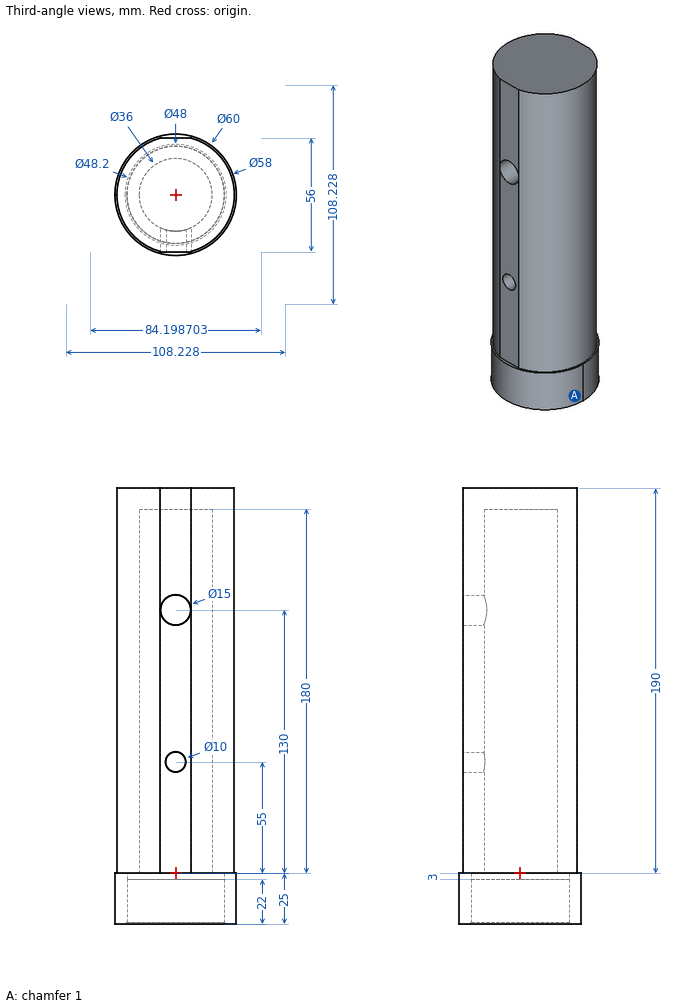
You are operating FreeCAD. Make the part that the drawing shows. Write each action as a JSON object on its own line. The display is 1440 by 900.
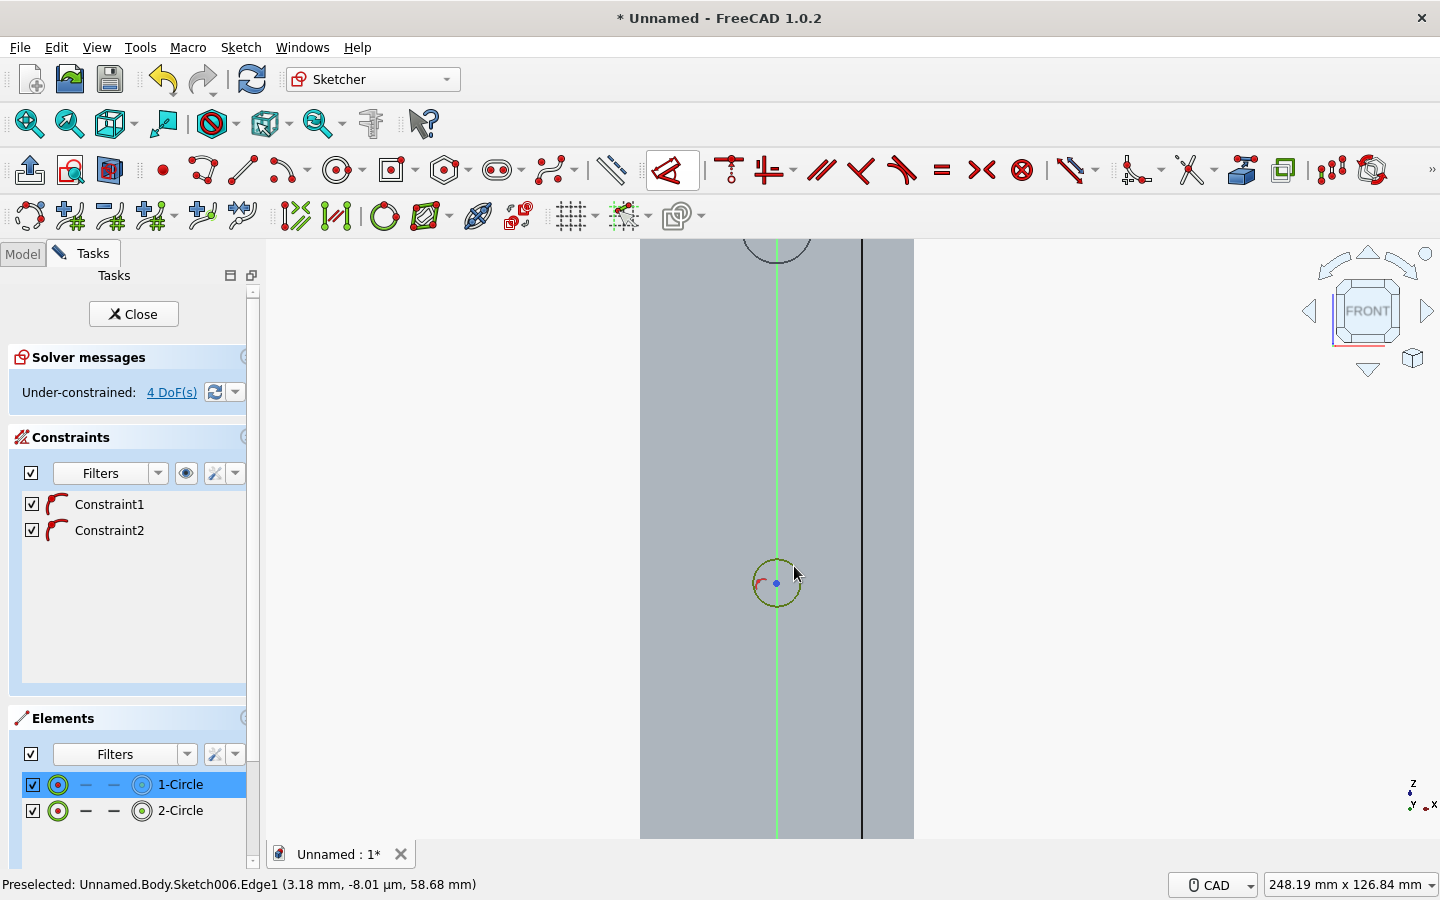
{"action": "key", "text": "k o"}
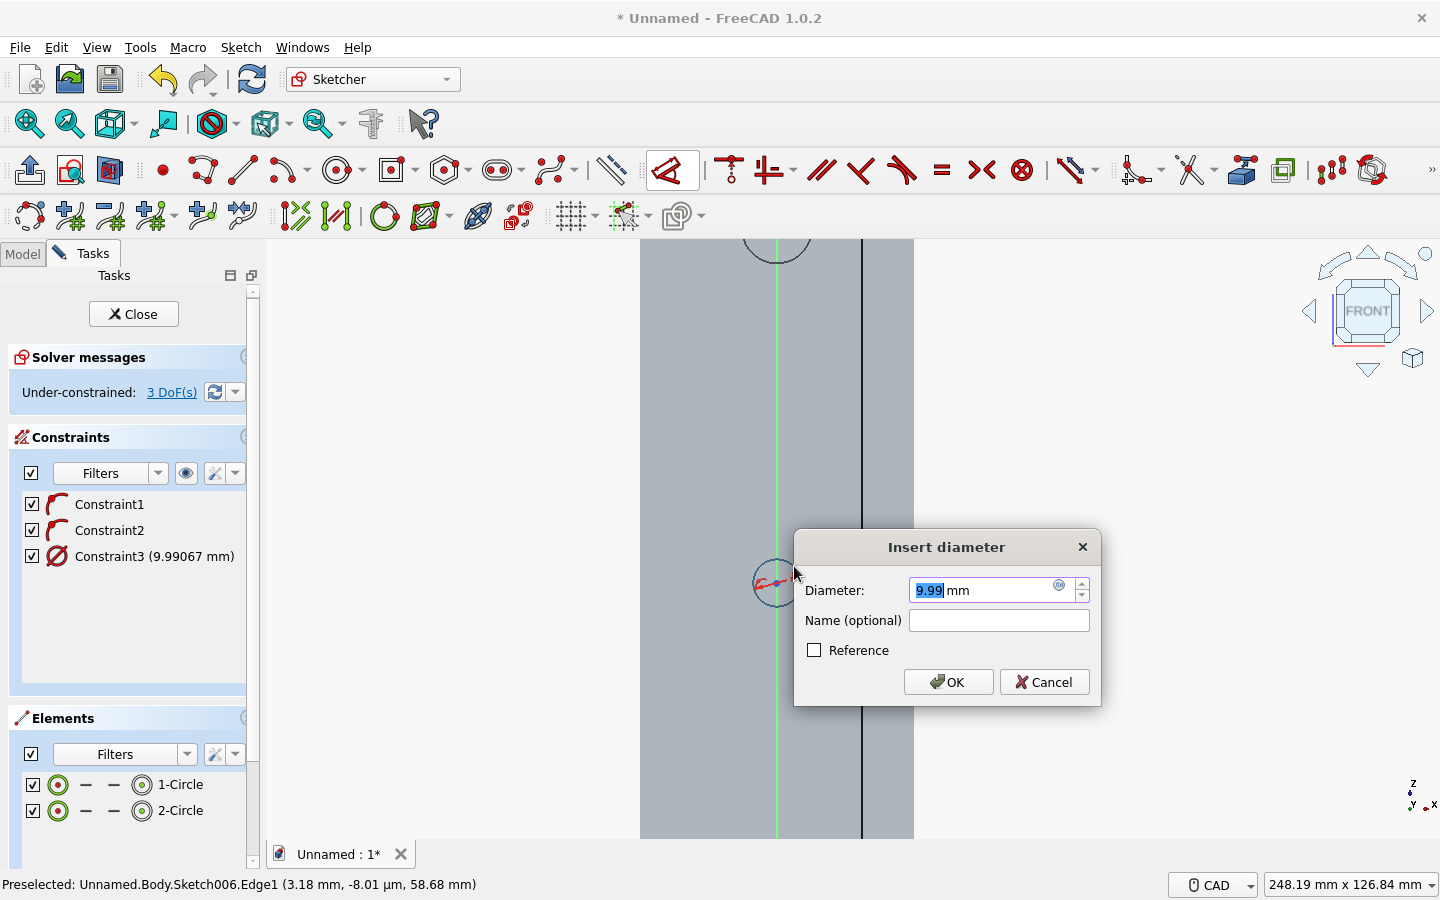
{"action": "type", "text": "10"}
{"action": "key", "text": "Return"}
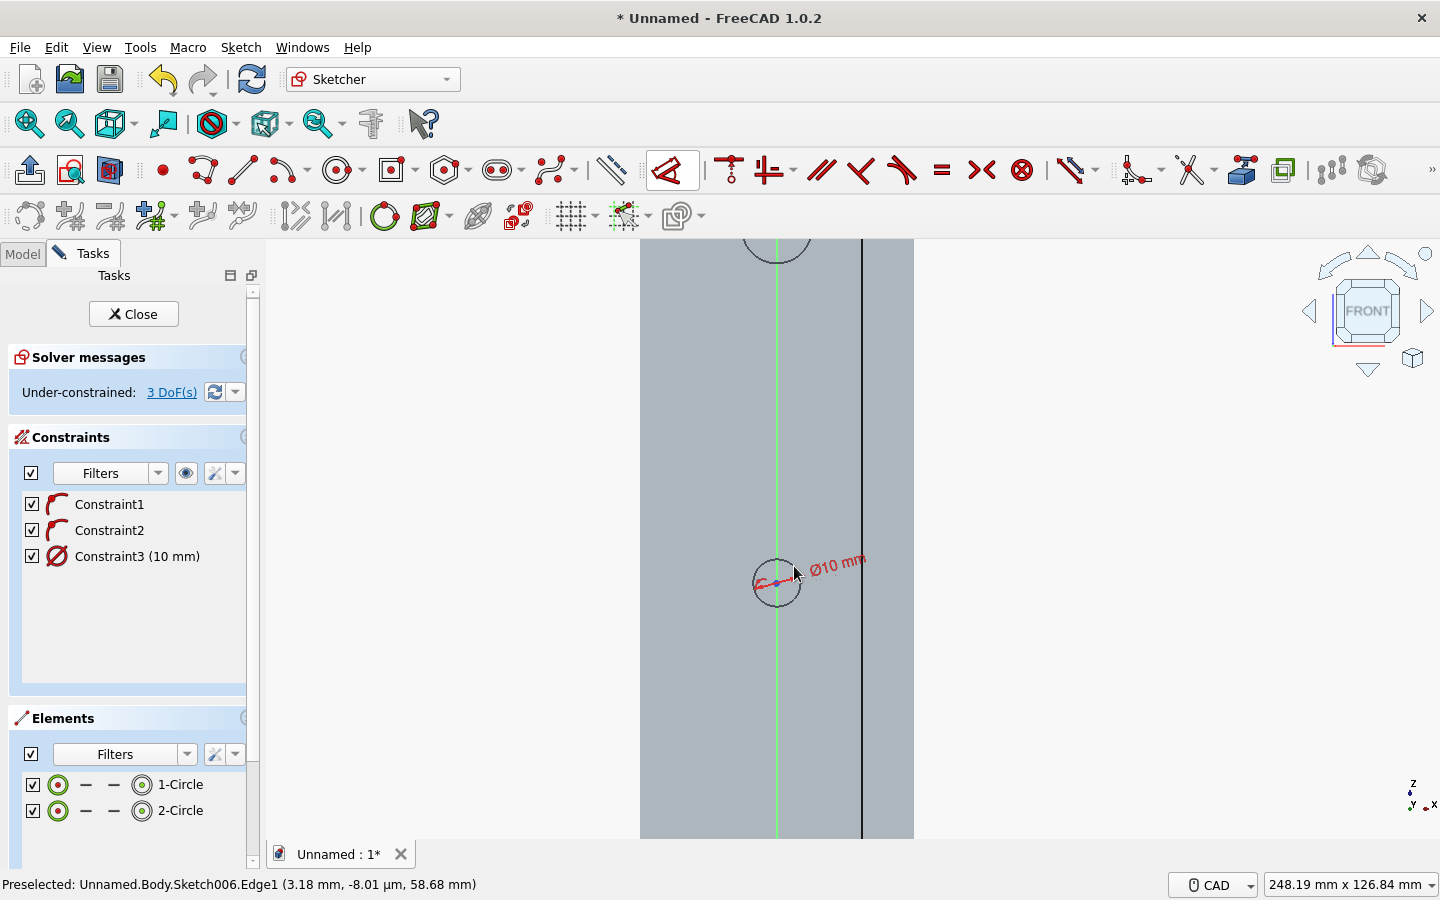
{"action": "scroll", "coordinate": [794, 566], "scroll_direction": "down", "scroll_amount": 3}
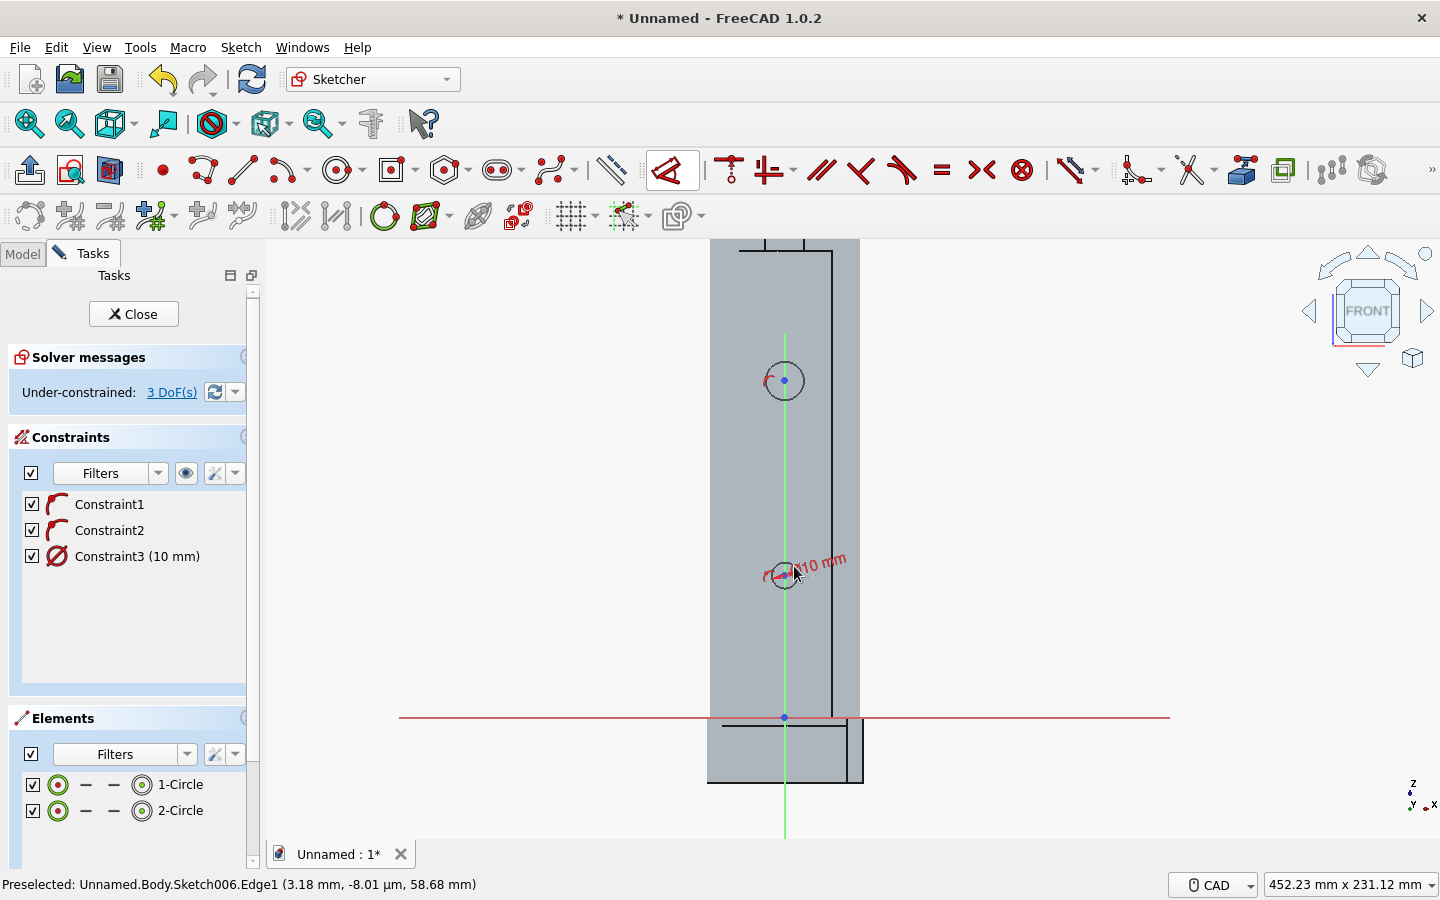
{"action": "left_click", "coordinate": [798, 367]}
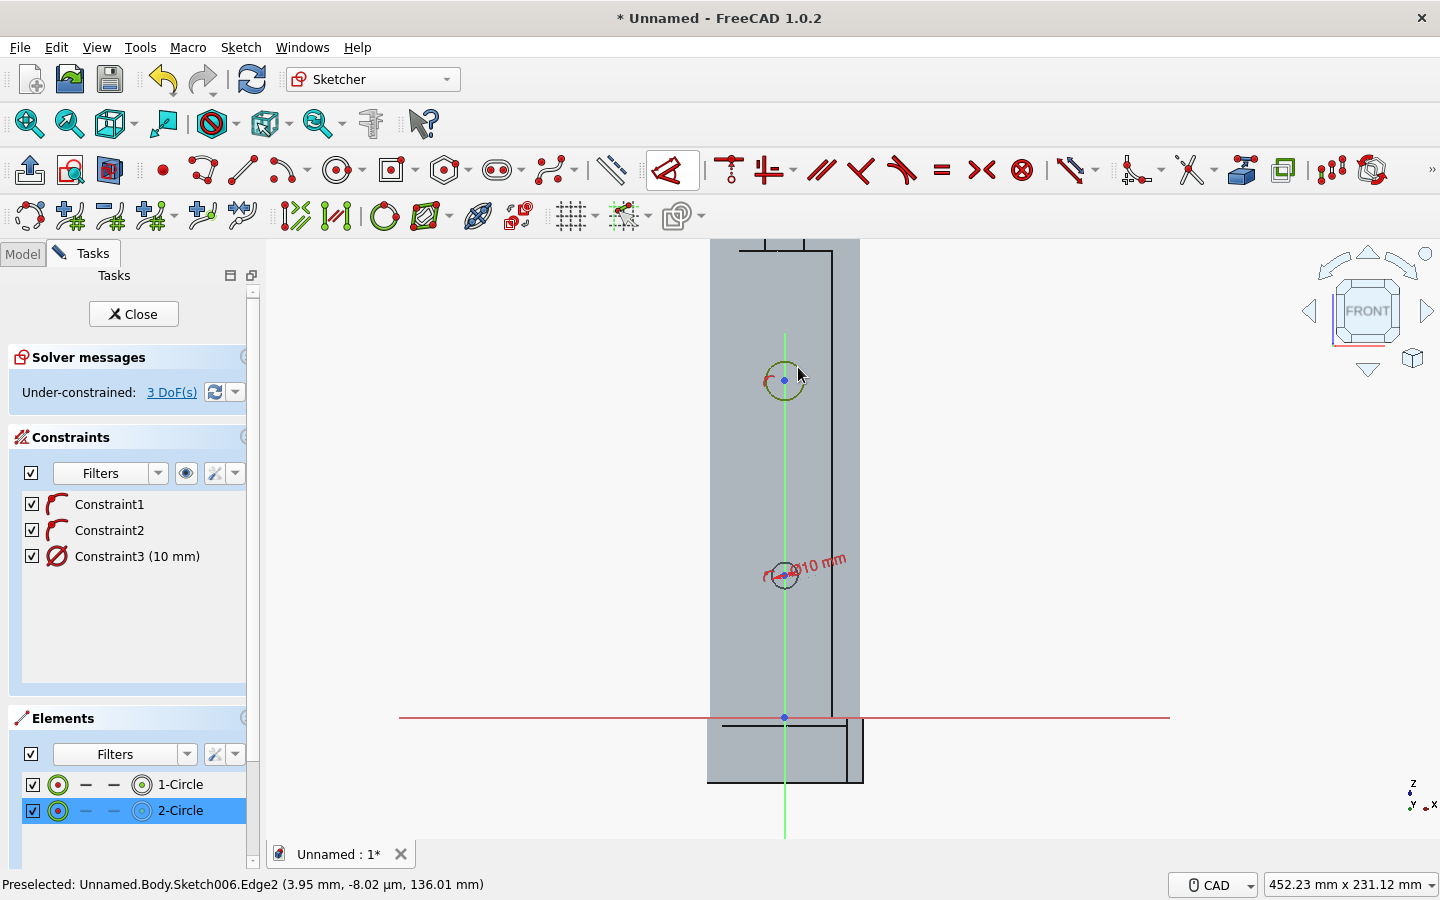
{"action": "key", "text": "k o"}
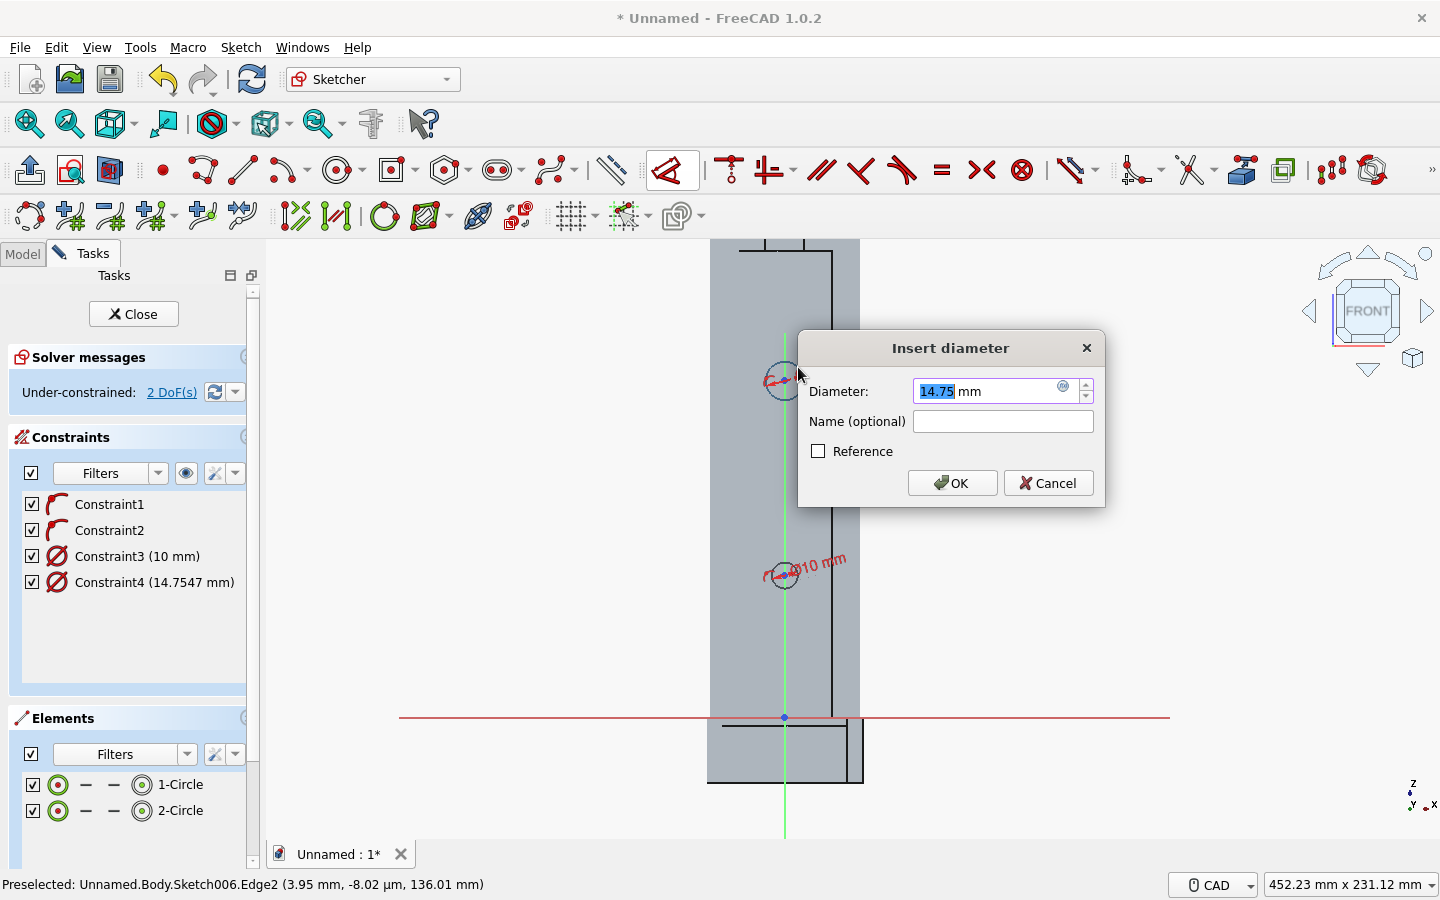
{"action": "type", "text": "15"}
{"action": "key", "text": "Return"}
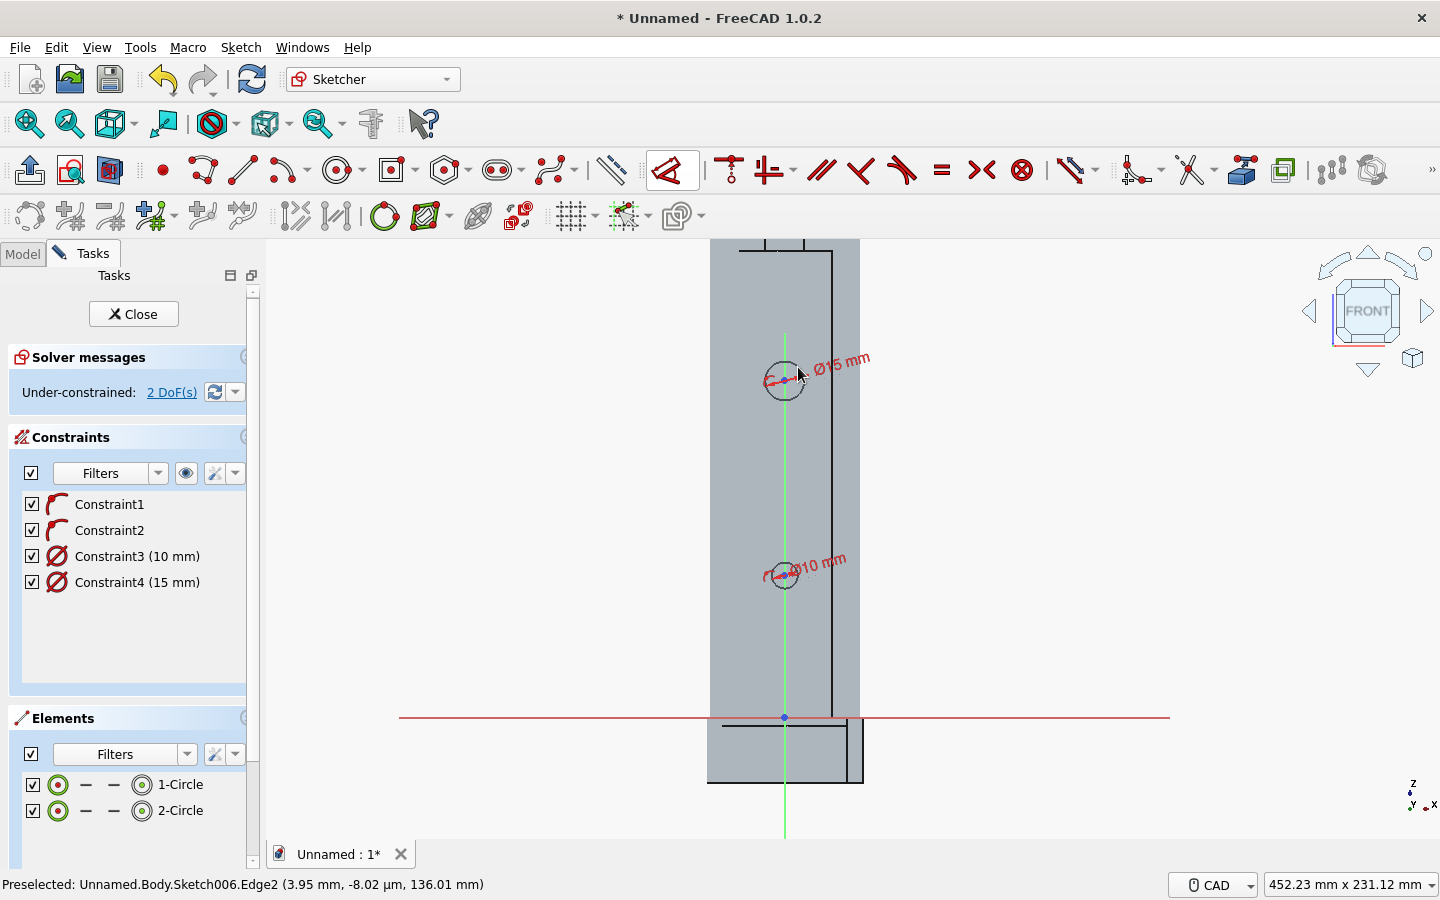
{"action": "left_click", "coordinate": [785, 576]}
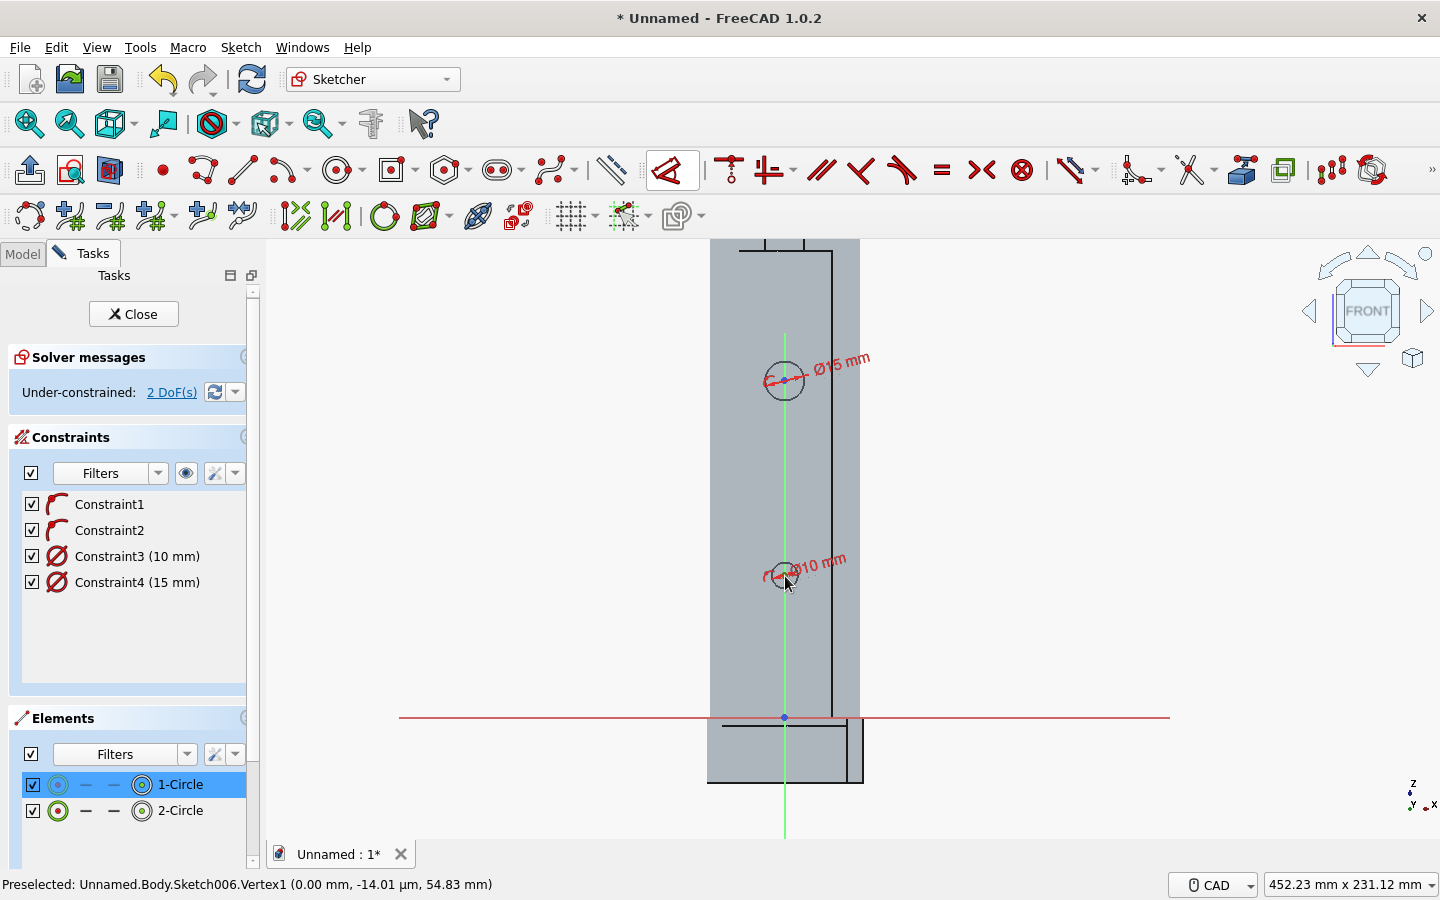
{"action": "left_click", "coordinate": [694, 170]}